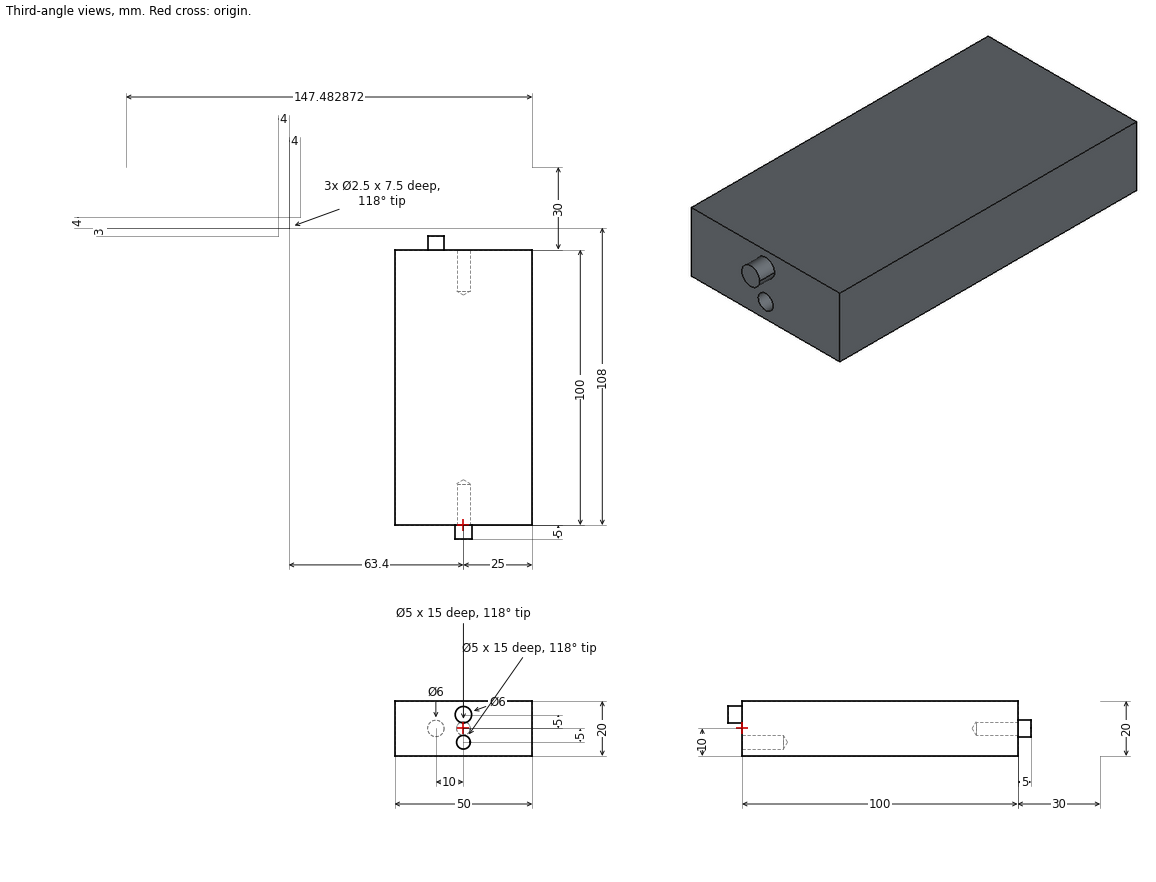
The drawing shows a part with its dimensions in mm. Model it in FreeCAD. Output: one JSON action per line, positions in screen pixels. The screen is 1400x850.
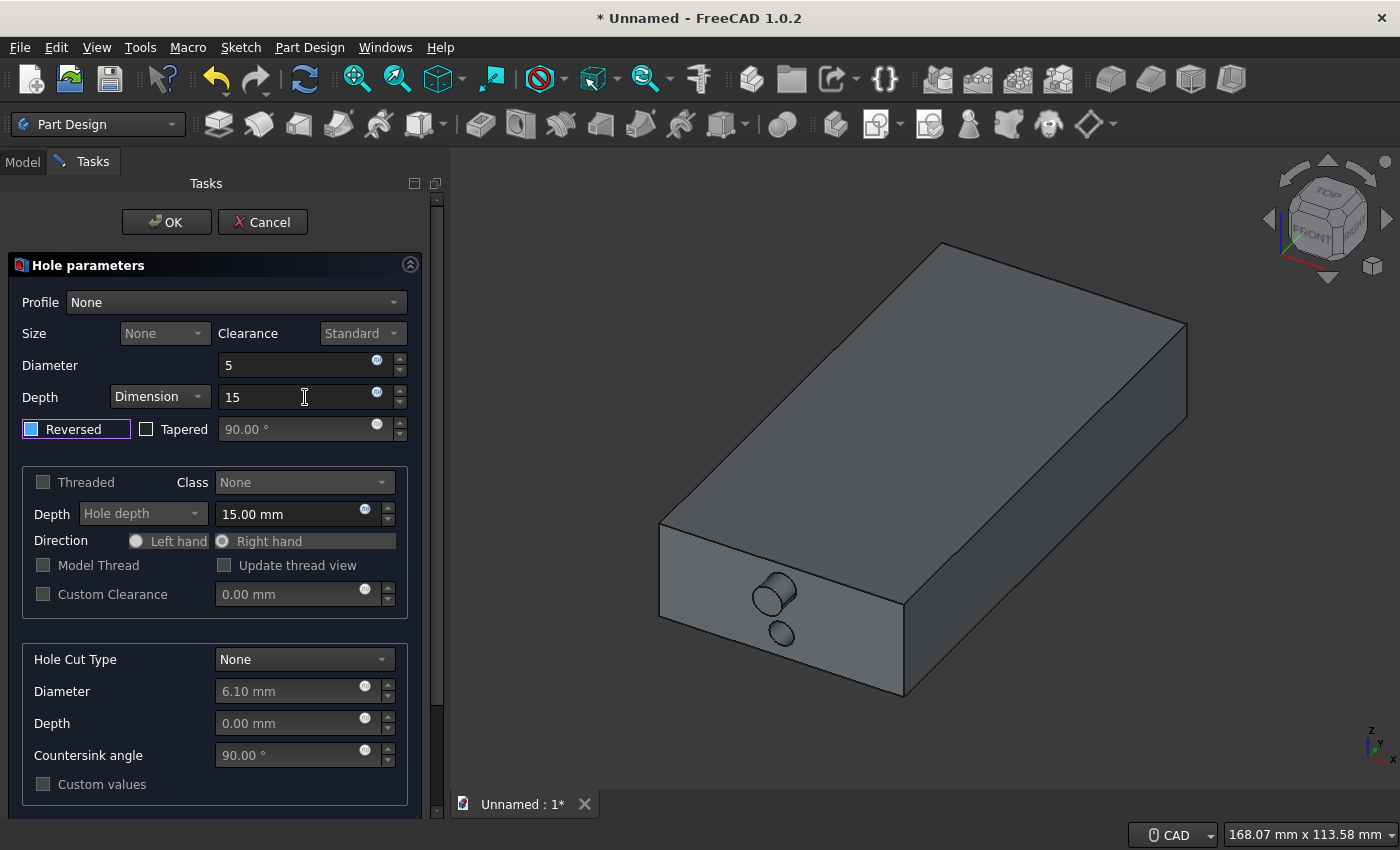
{"action": "left_click", "coordinate": [167, 222]}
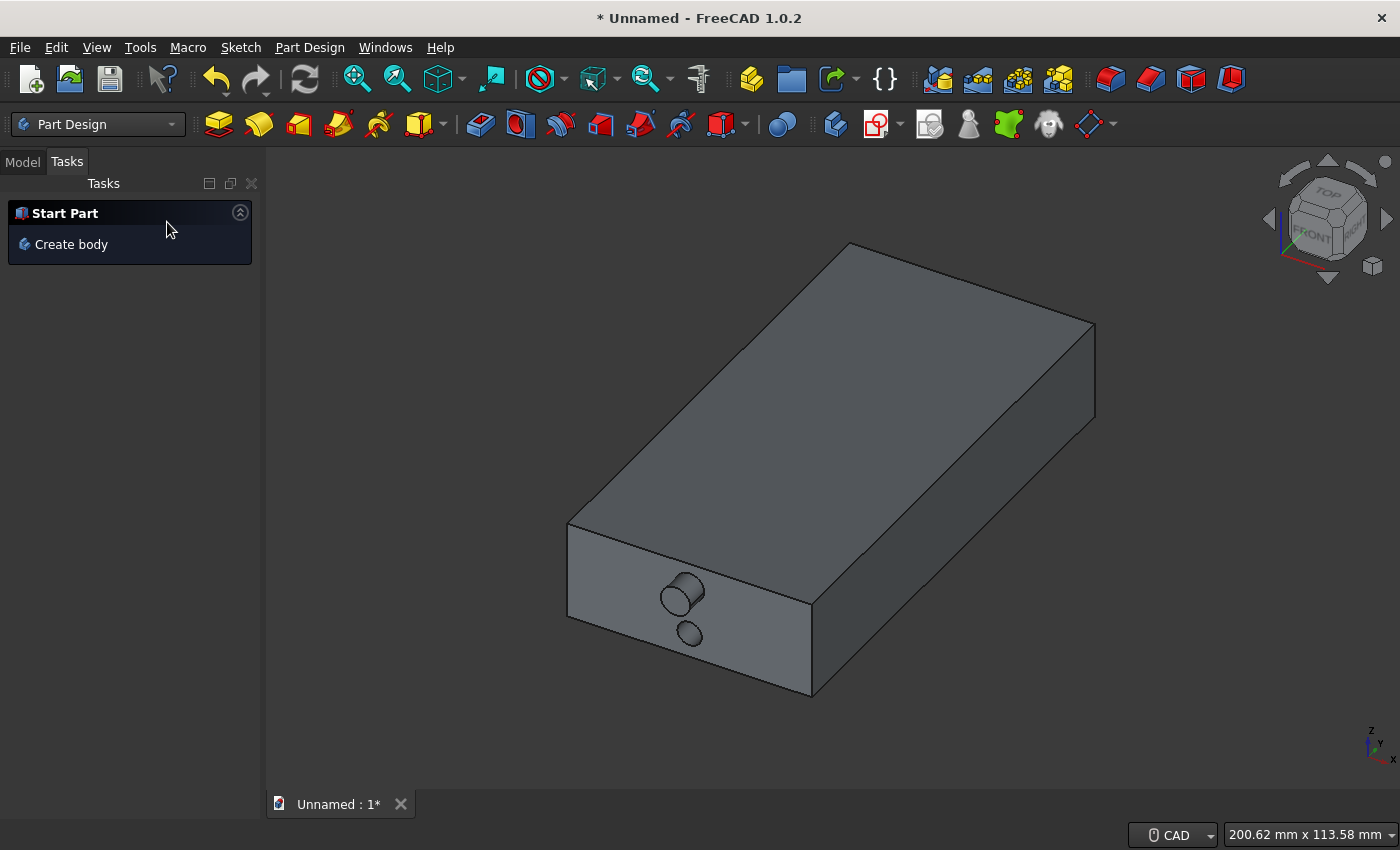
{"action": "left_click", "coordinate": [1034, 429]}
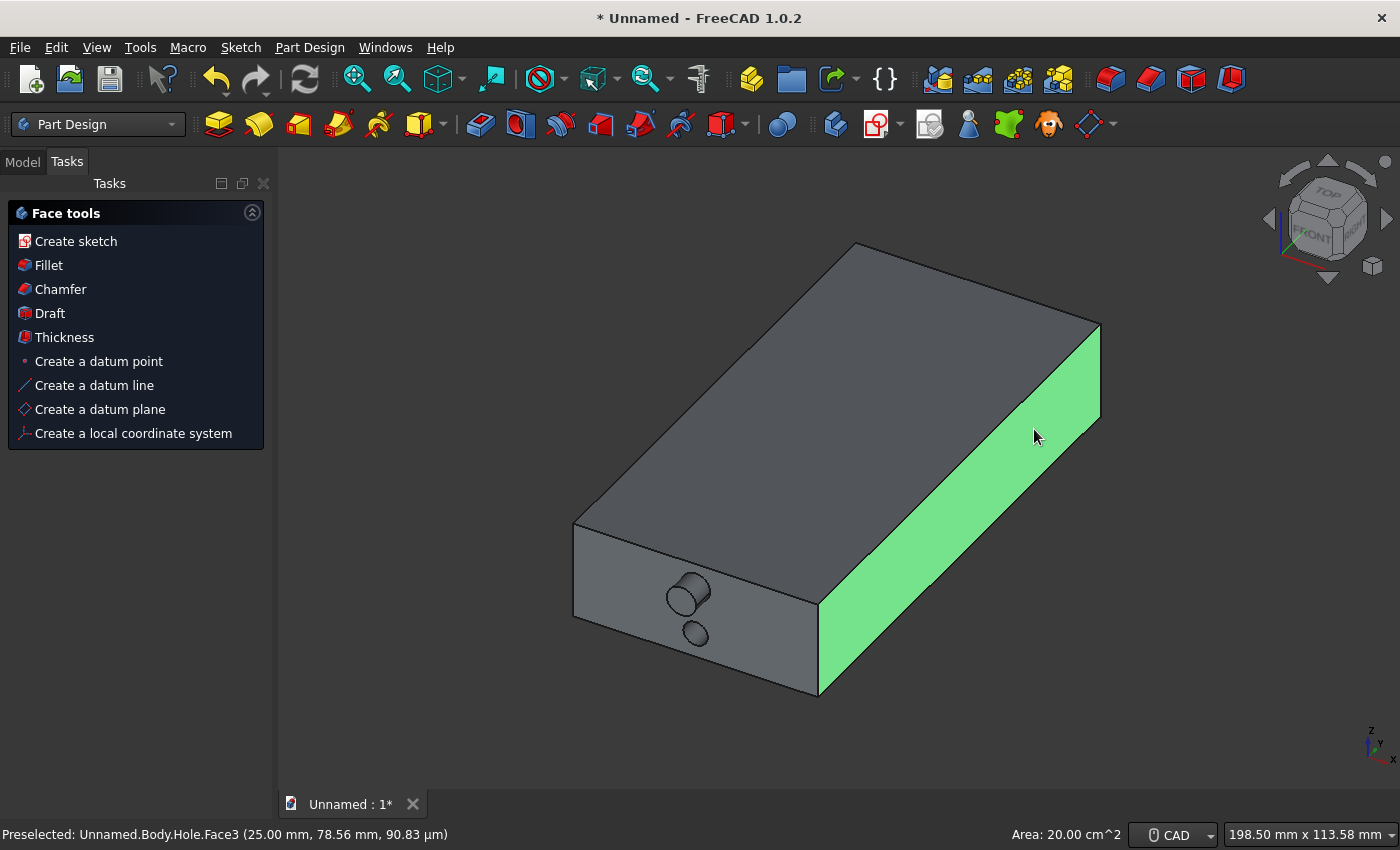
{"action": "left_click", "coordinate": [876, 124]}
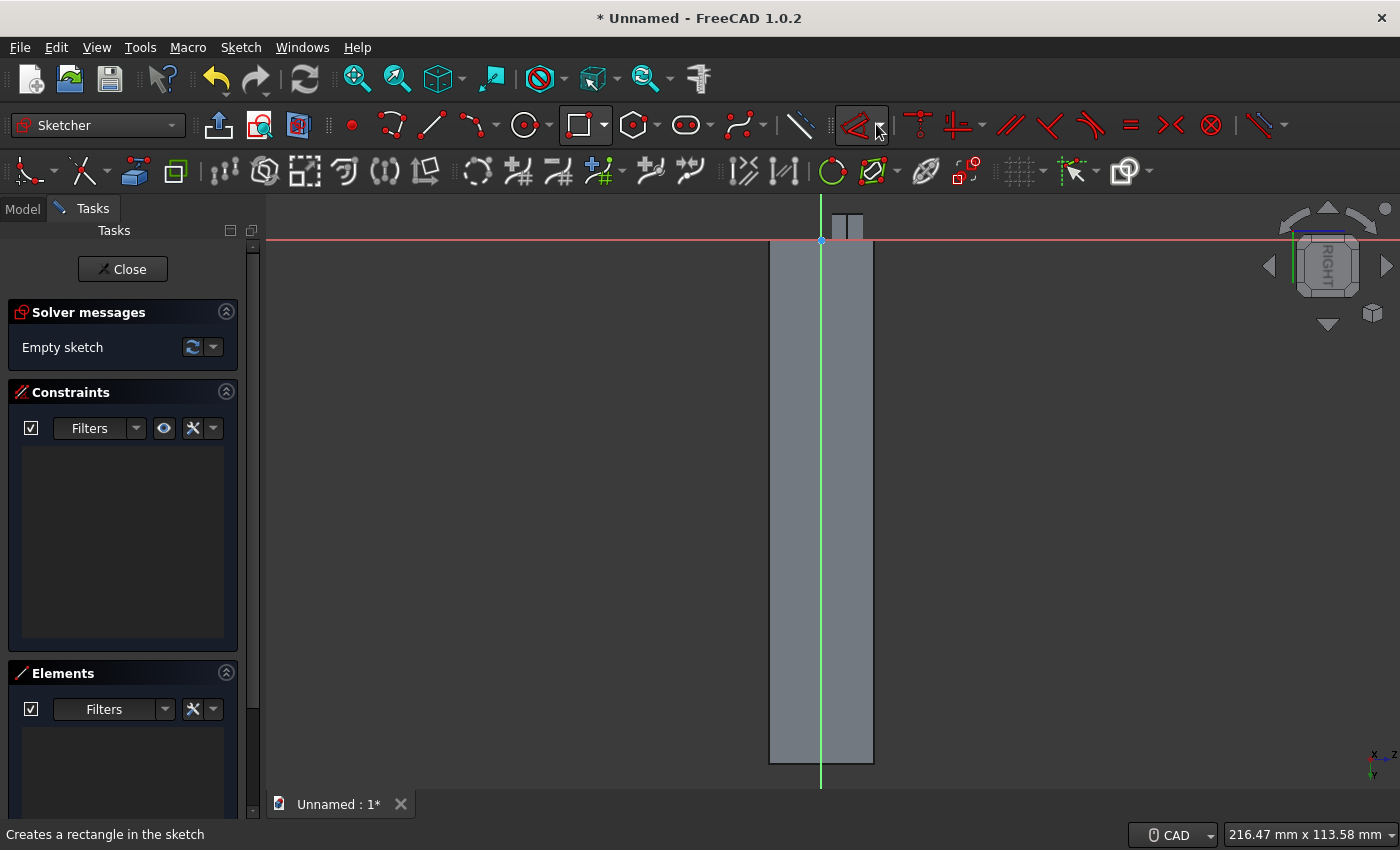
{"action": "scroll", "coordinate": [764, 492], "scroll_direction": "down", "scroll_amount": 5}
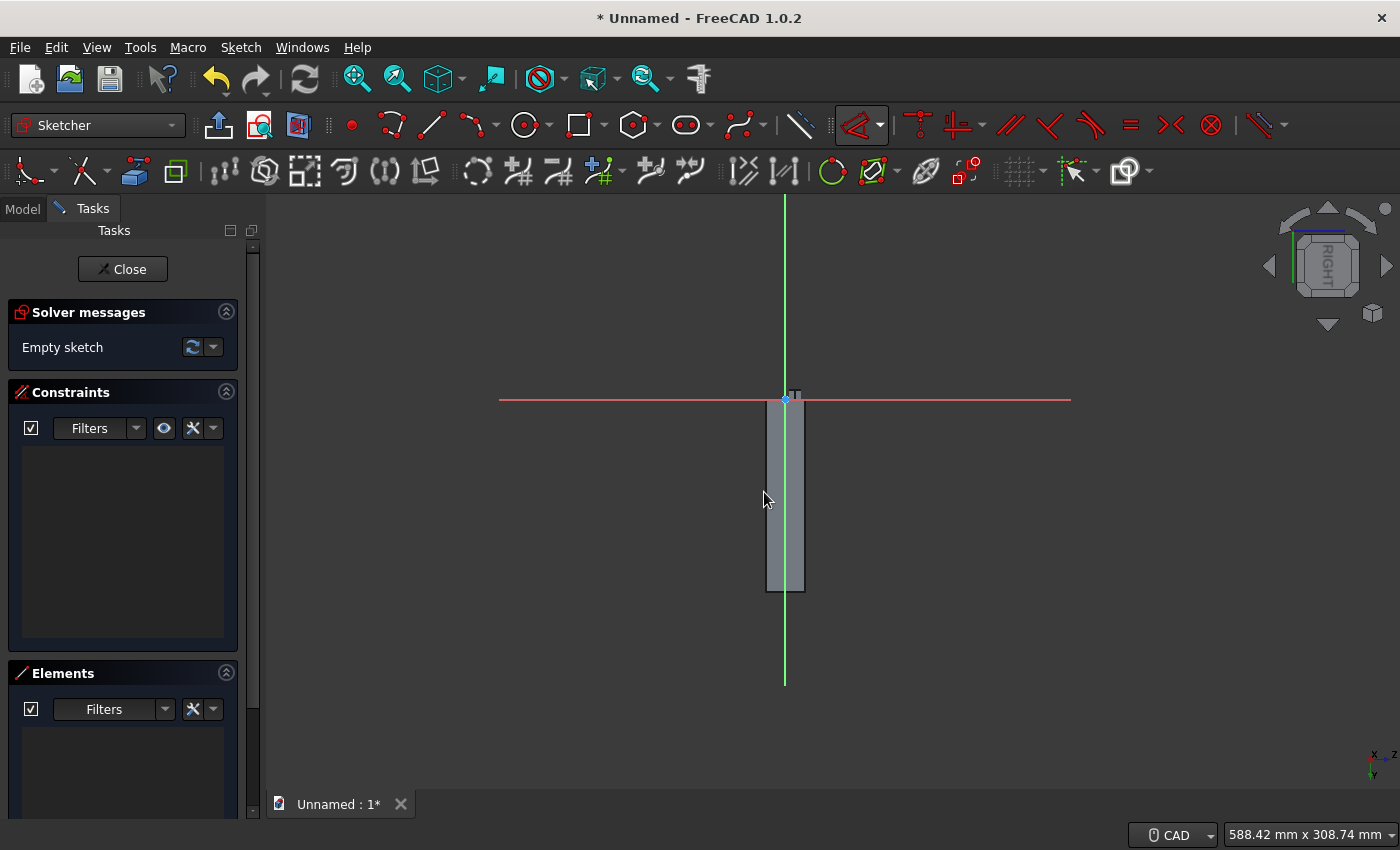
{"action": "scroll", "coordinate": [789, 647], "scroll_direction": "up", "scroll_amount": 9}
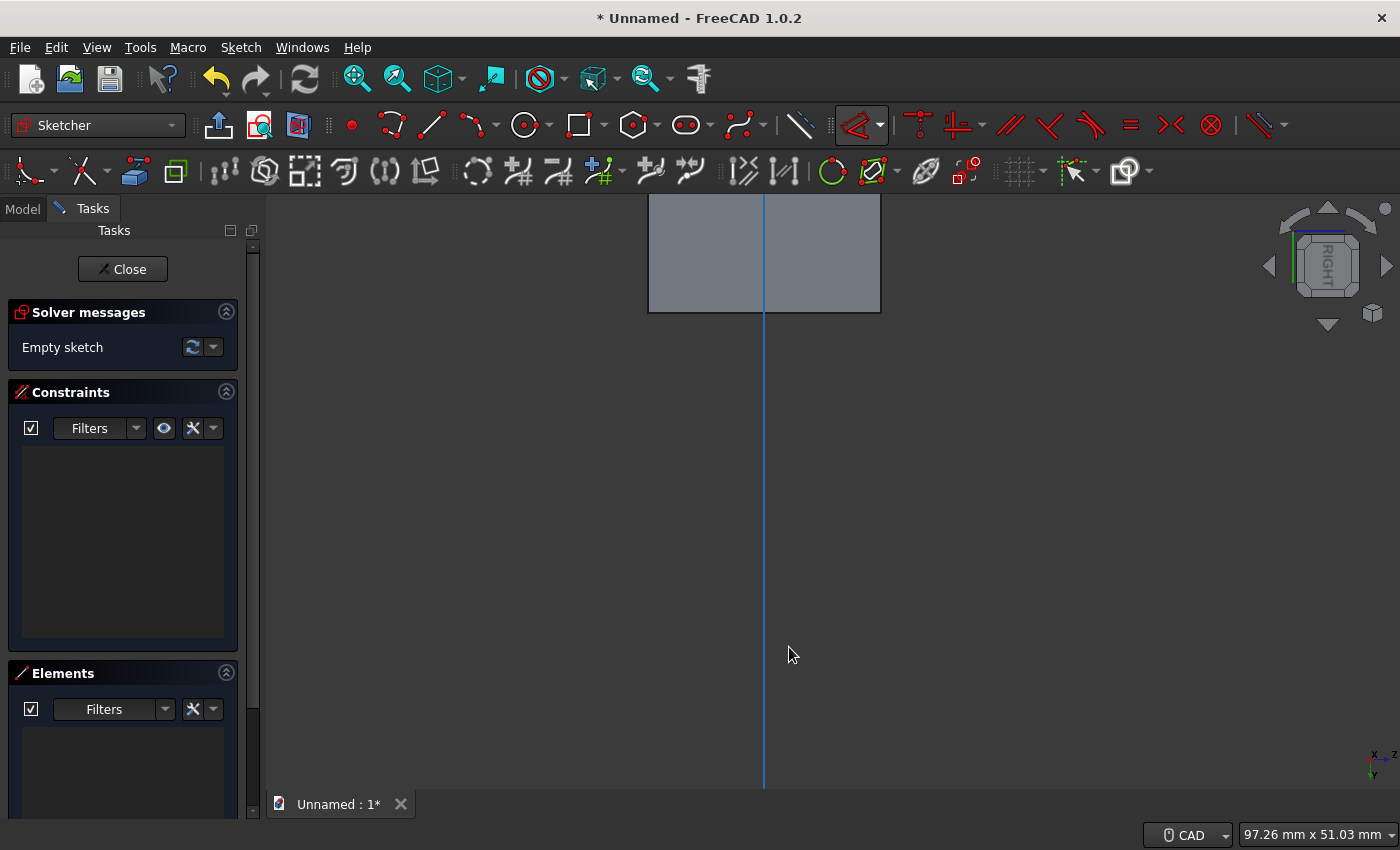
{"action": "left_click", "coordinate": [580, 126]}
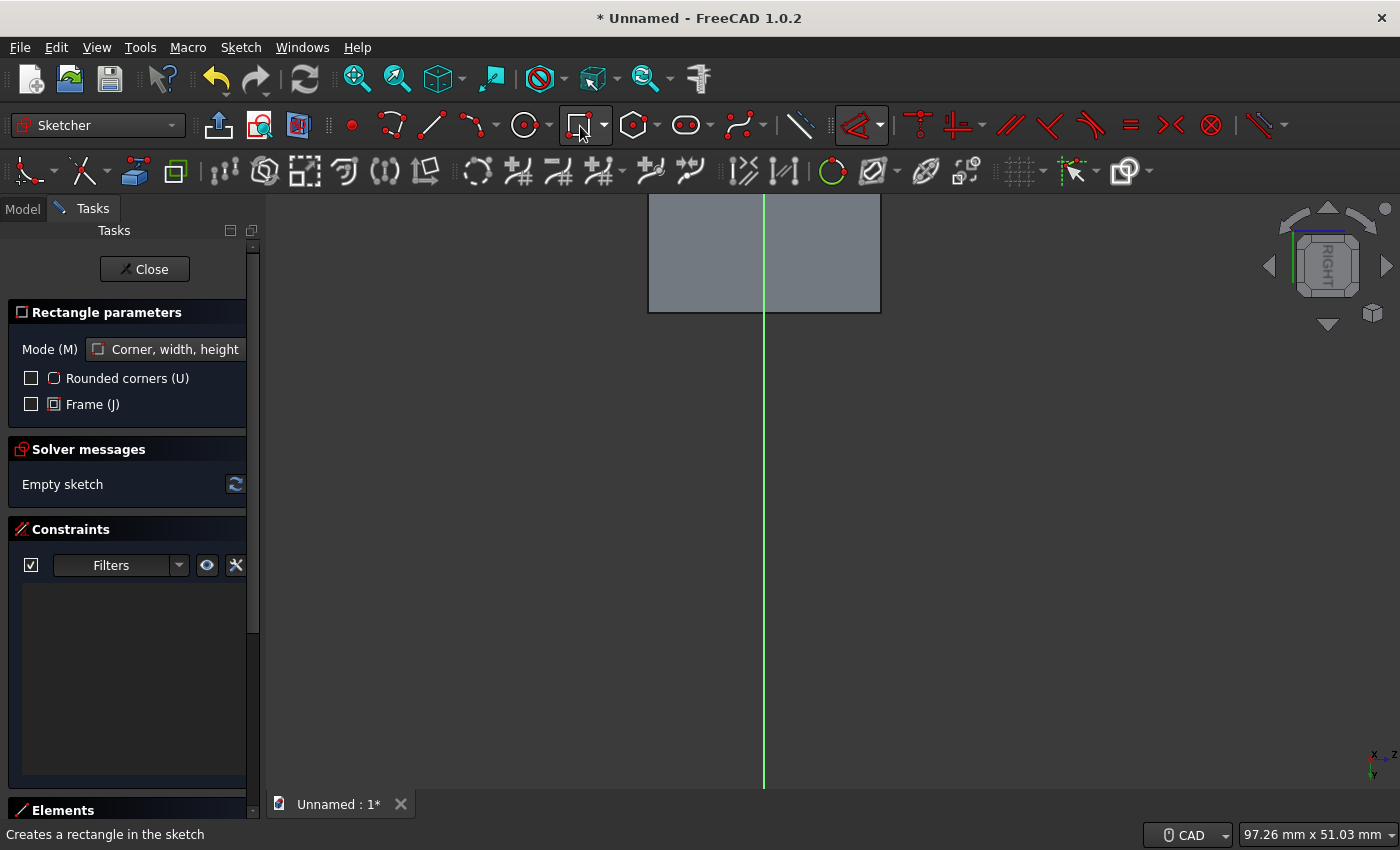
{"action": "left_click", "coordinate": [648, 313]}
{"action": "left_click", "coordinate": [881, 663]}
{"action": "key", "text": "Escape"}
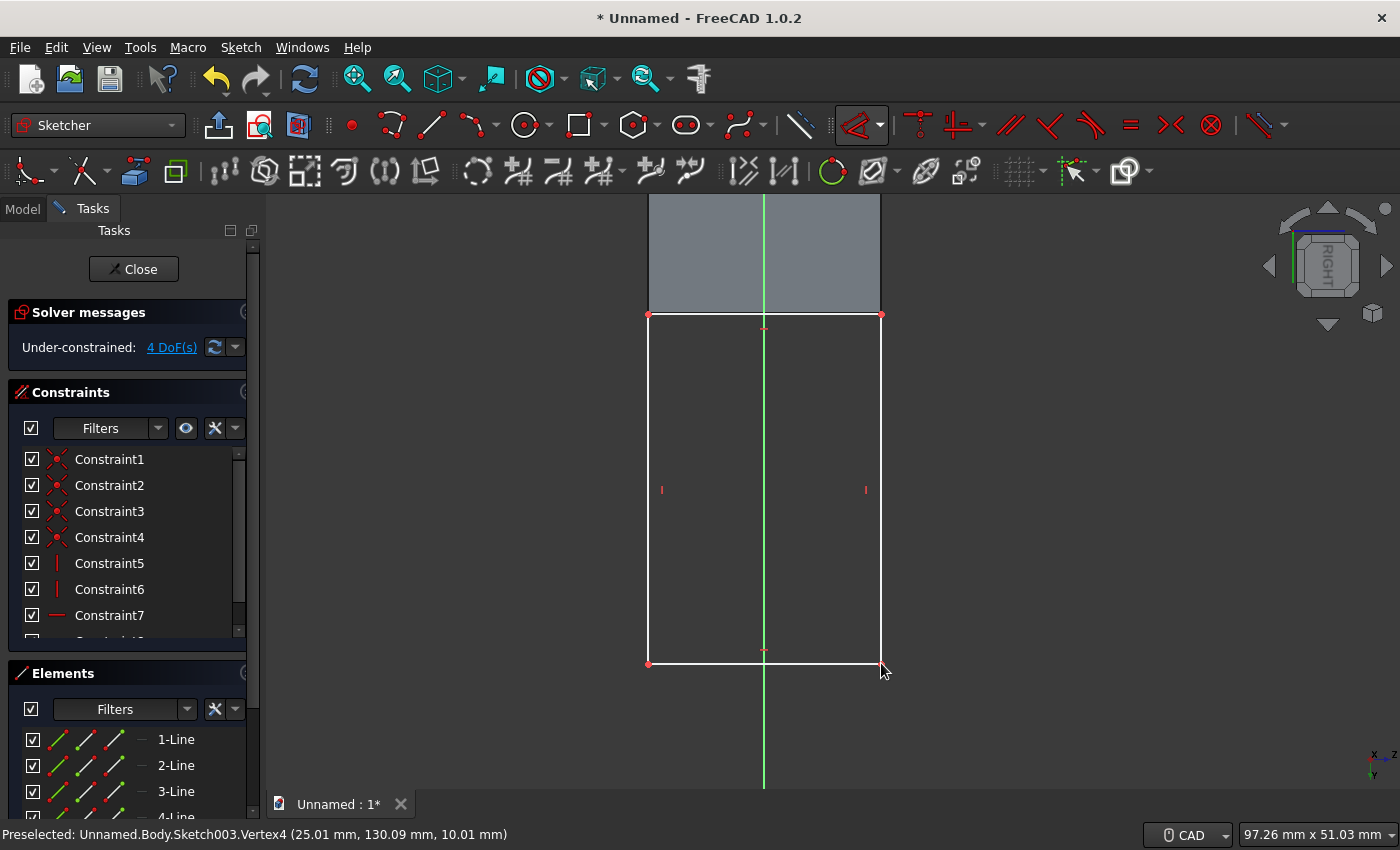
{"action": "left_click", "coordinate": [648, 419]}